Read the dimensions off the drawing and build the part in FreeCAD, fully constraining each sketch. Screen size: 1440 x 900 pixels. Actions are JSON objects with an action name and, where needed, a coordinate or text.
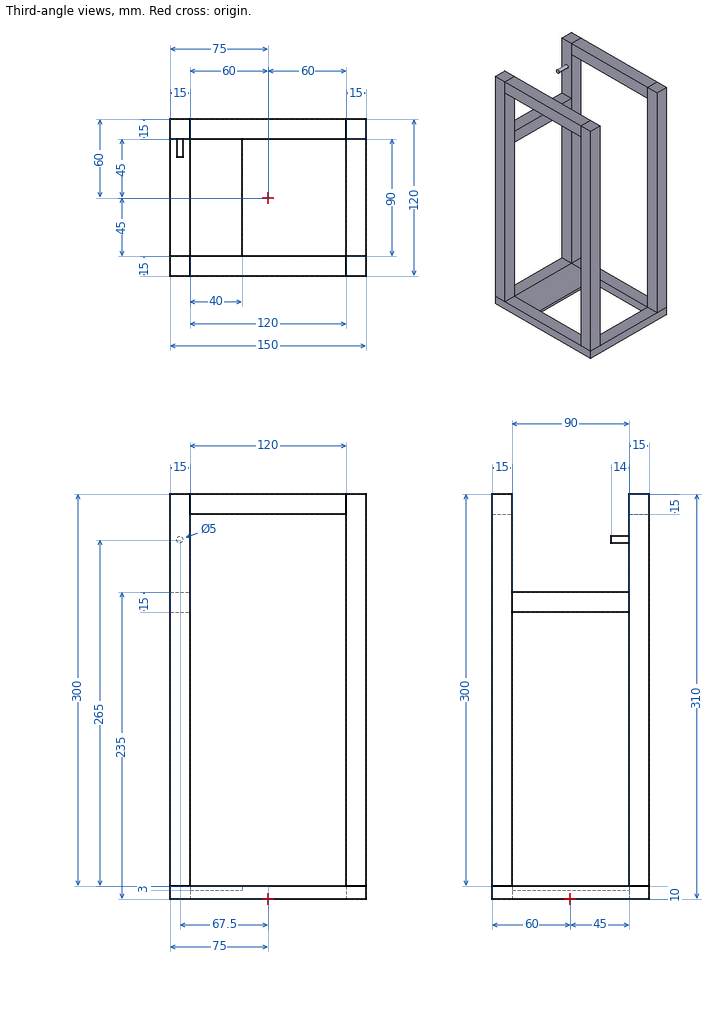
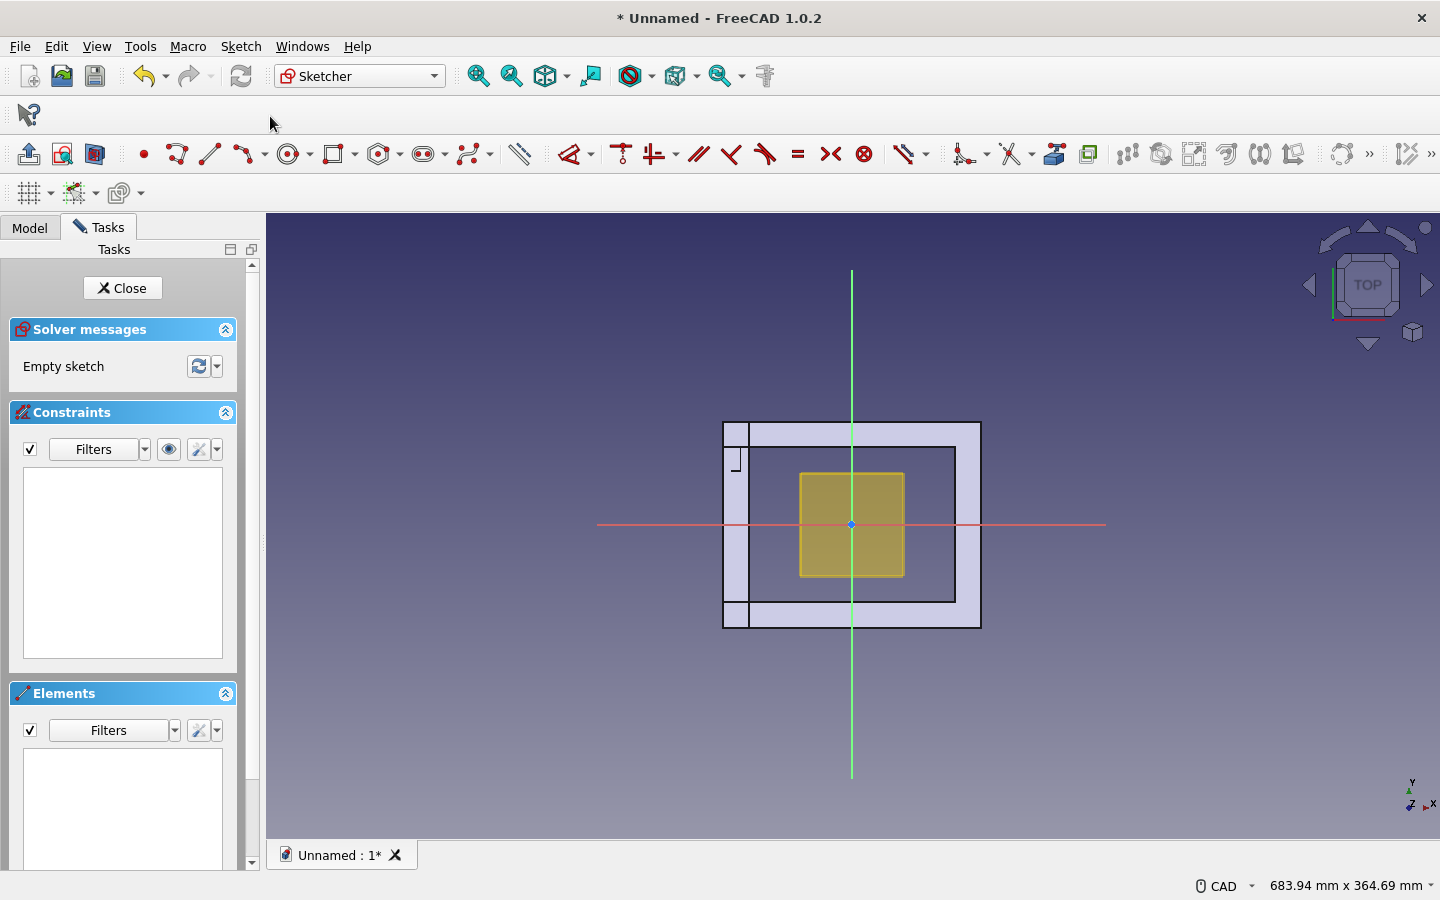
{"action": "scroll", "coordinate": [980, 429], "scroll_direction": "up", "scroll_amount": 14}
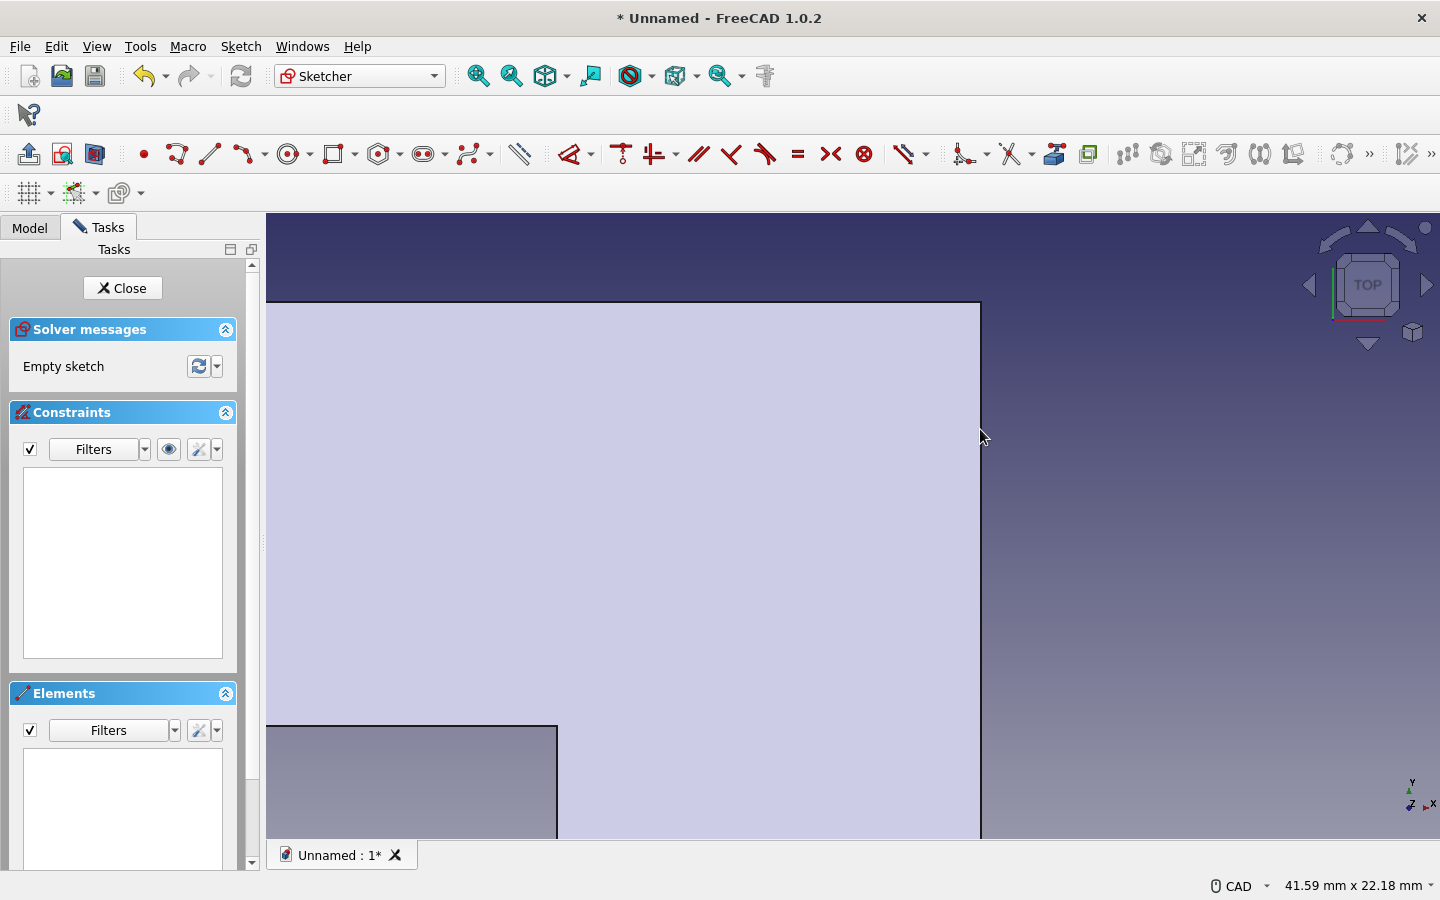
{"action": "left_click", "coordinate": [332, 154]}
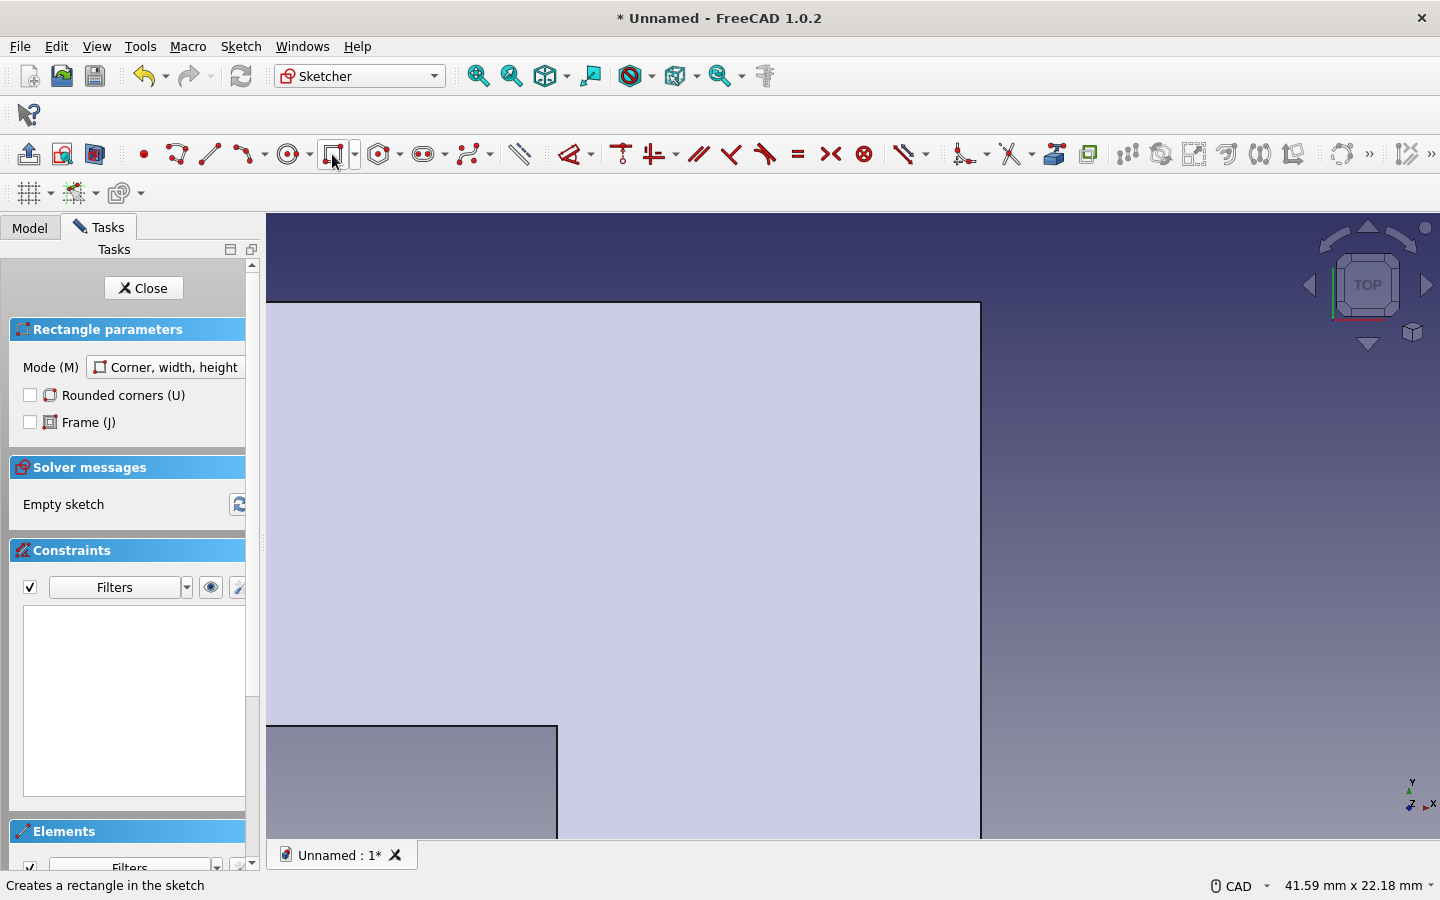
{"action": "left_click", "coordinate": [557, 302]}
{"action": "left_click", "coordinate": [981, 726]}
{"action": "key", "text": "Escape"}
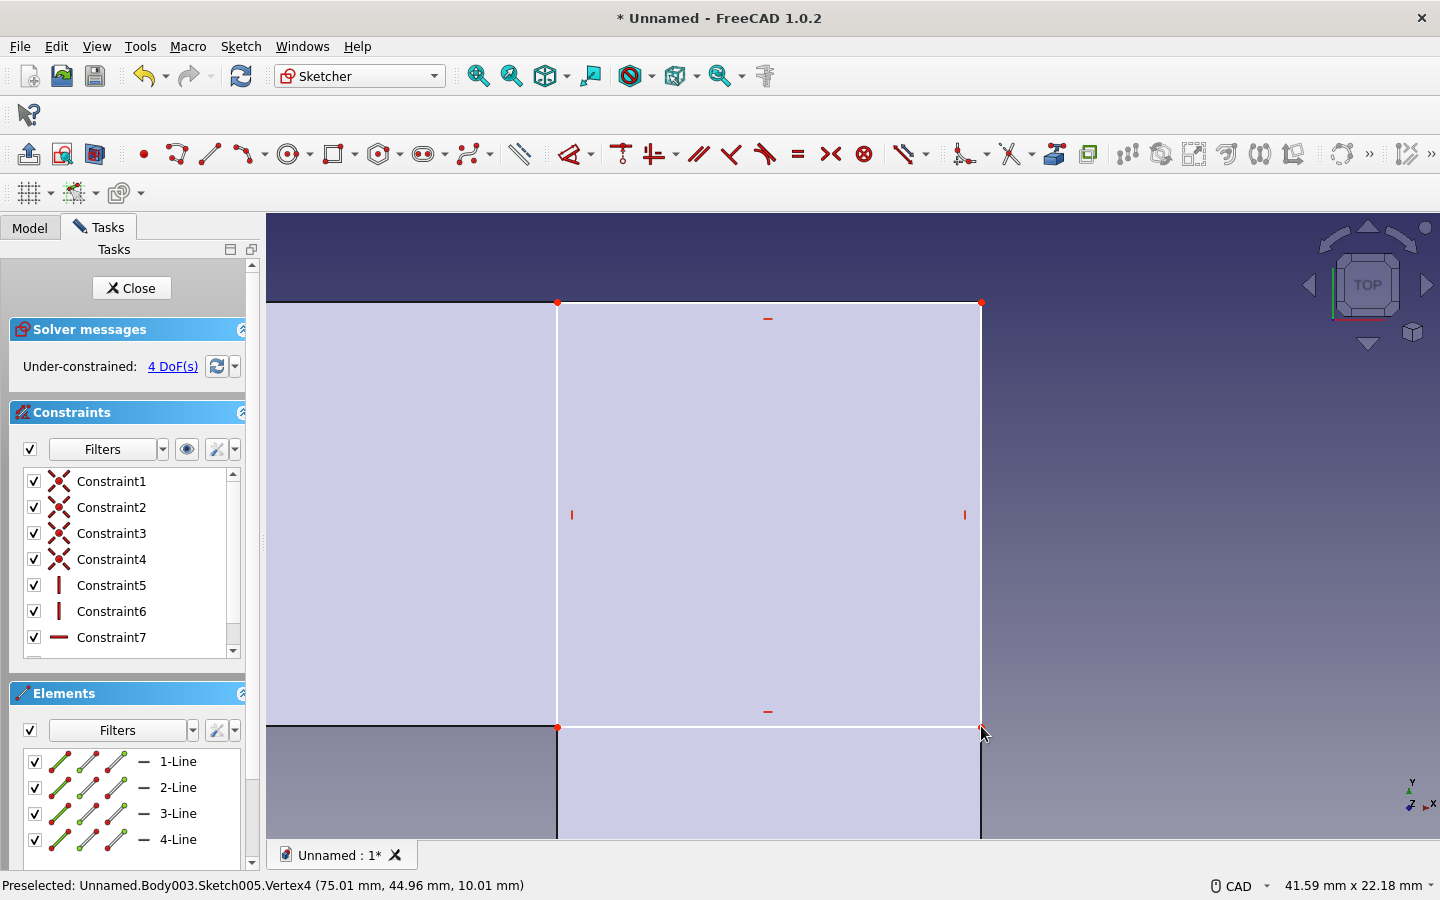
{"action": "left_click", "coordinate": [568, 154]}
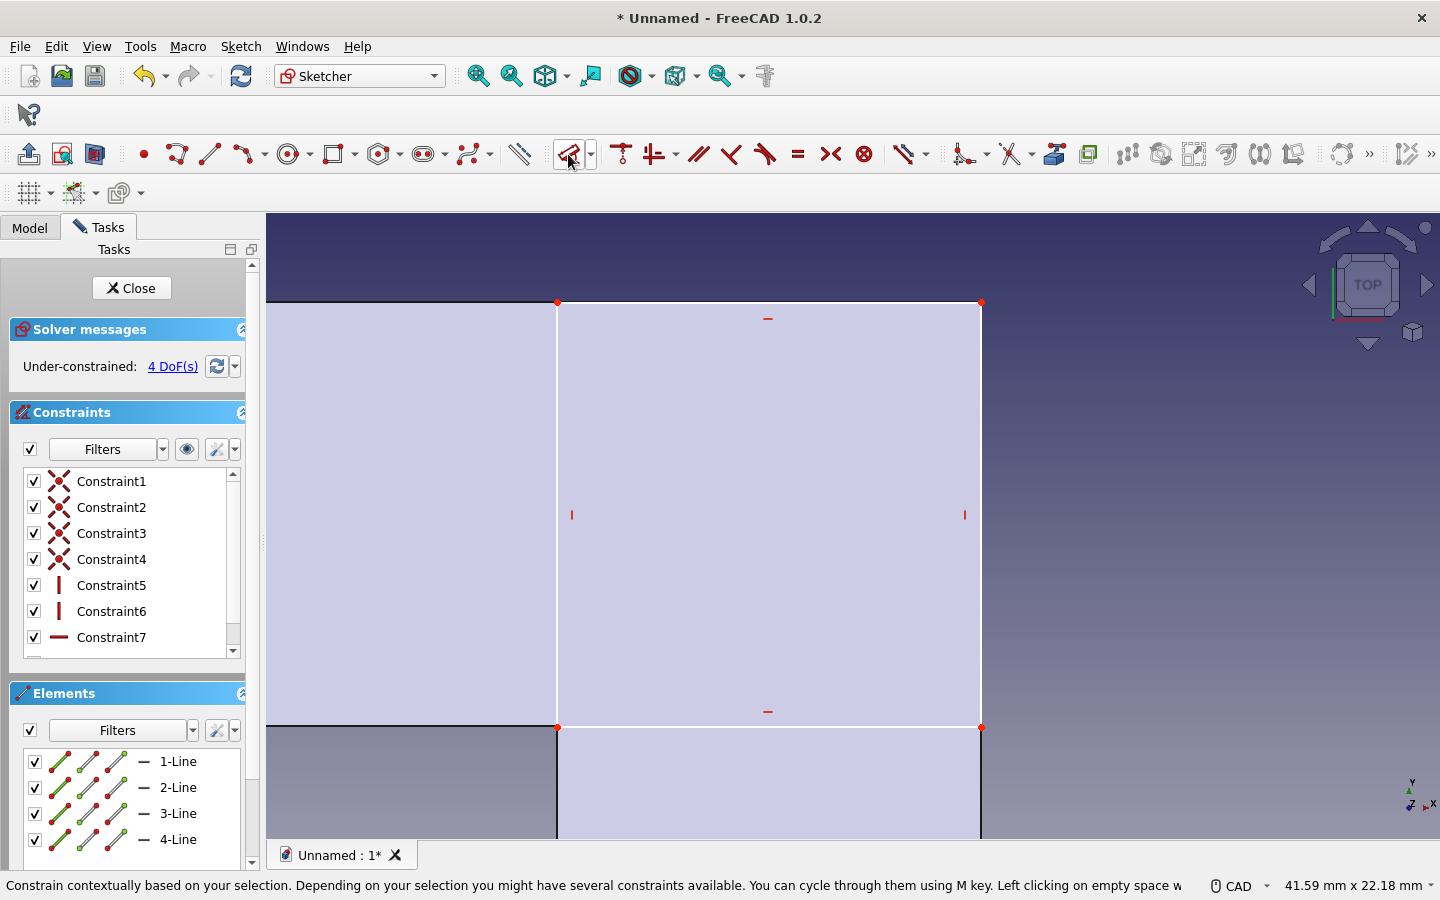
{"action": "left_click", "coordinate": [557, 430]}
{"action": "left_click", "coordinate": [523, 515]}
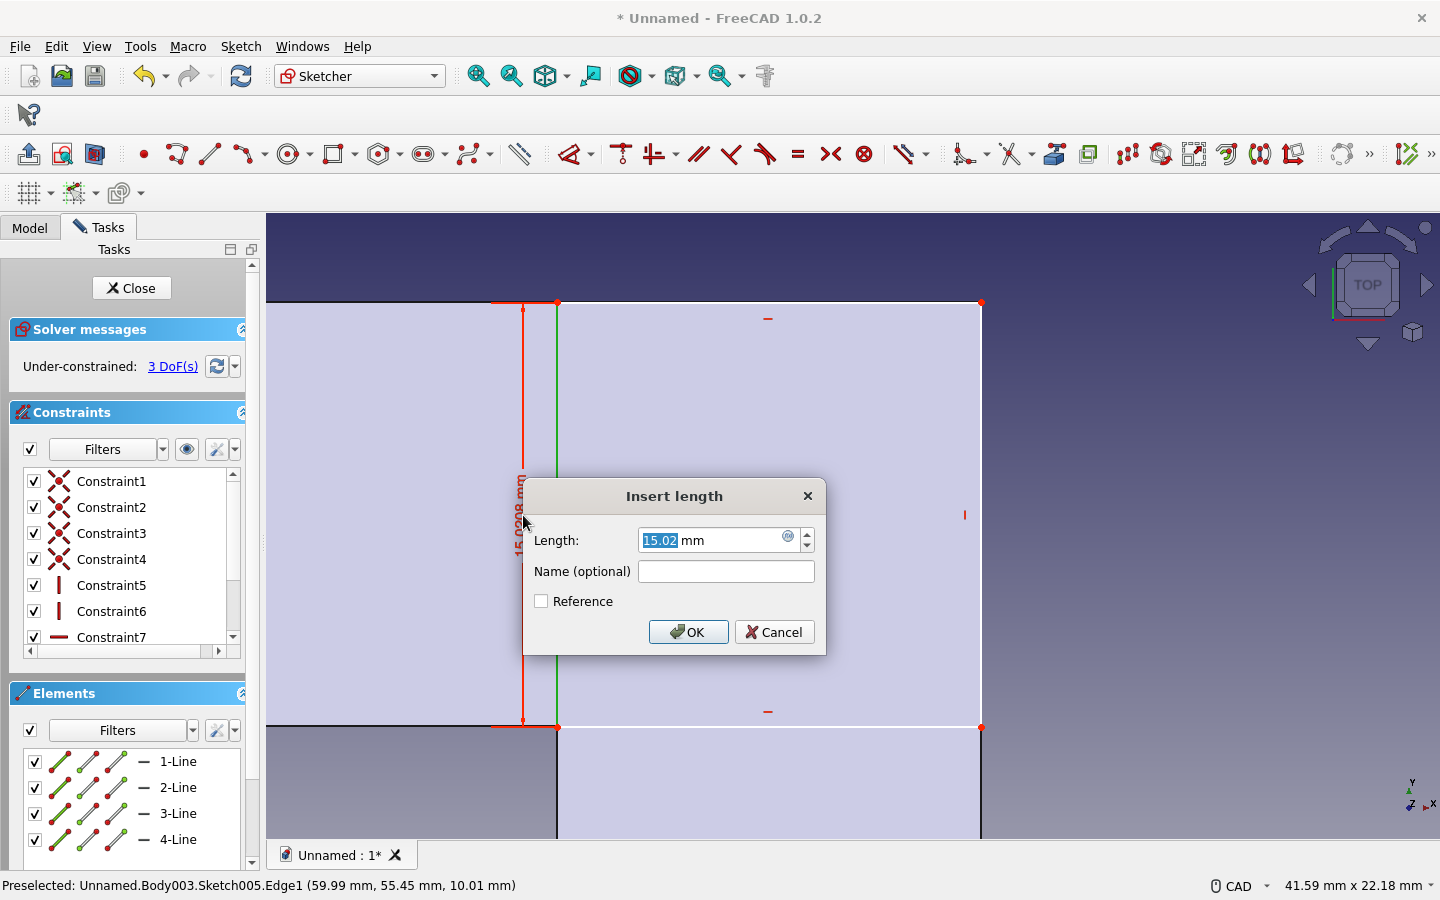
{"action": "type", "text": "15"}
{"action": "key", "text": "Return"}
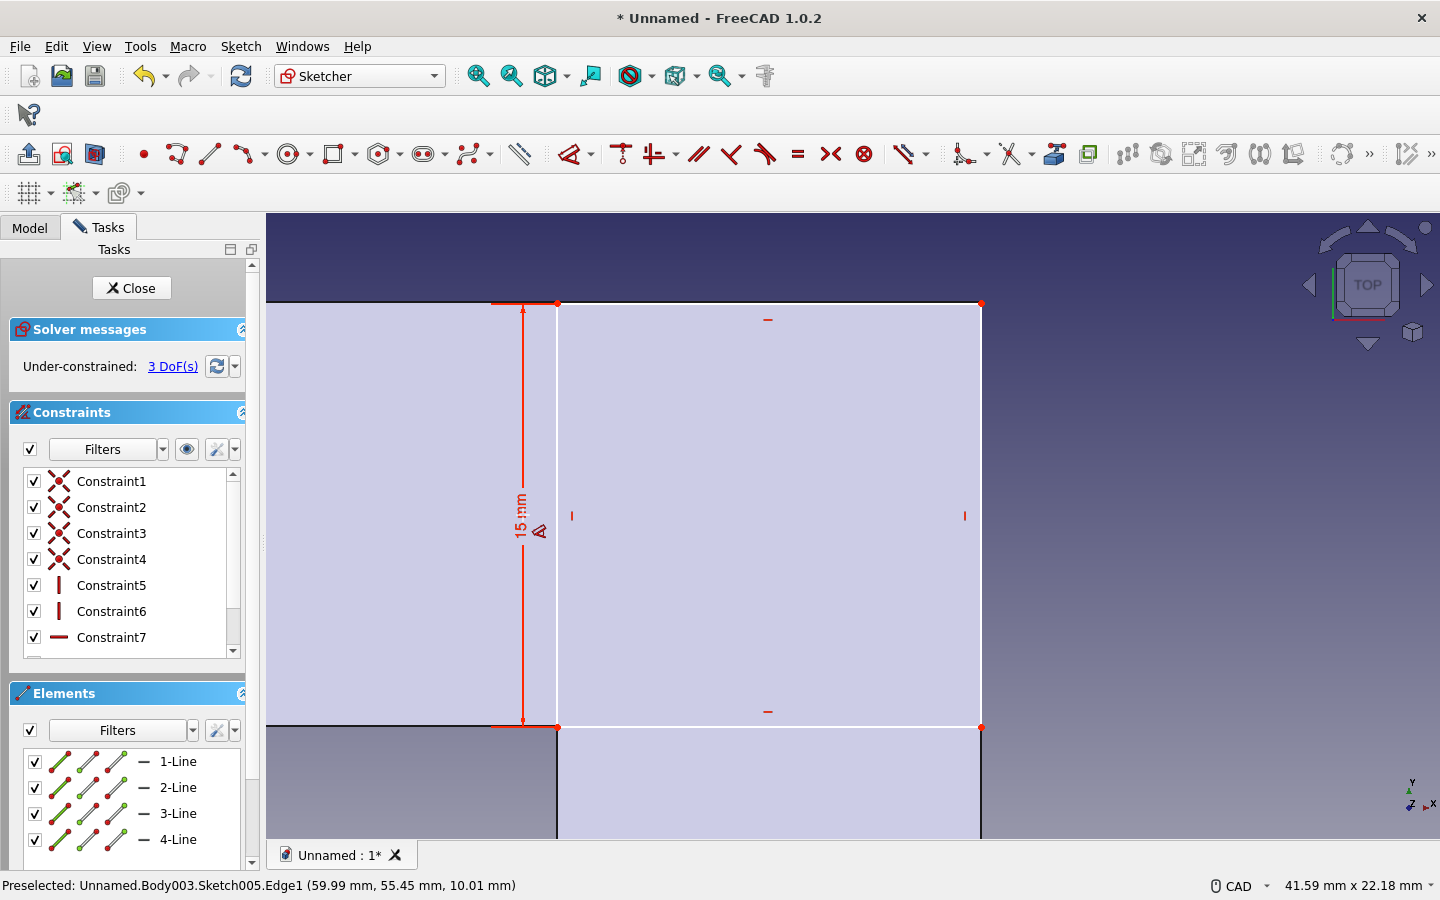
{"action": "left_click", "coordinate": [684, 727]}
{"action": "left_click", "coordinate": [769, 761]}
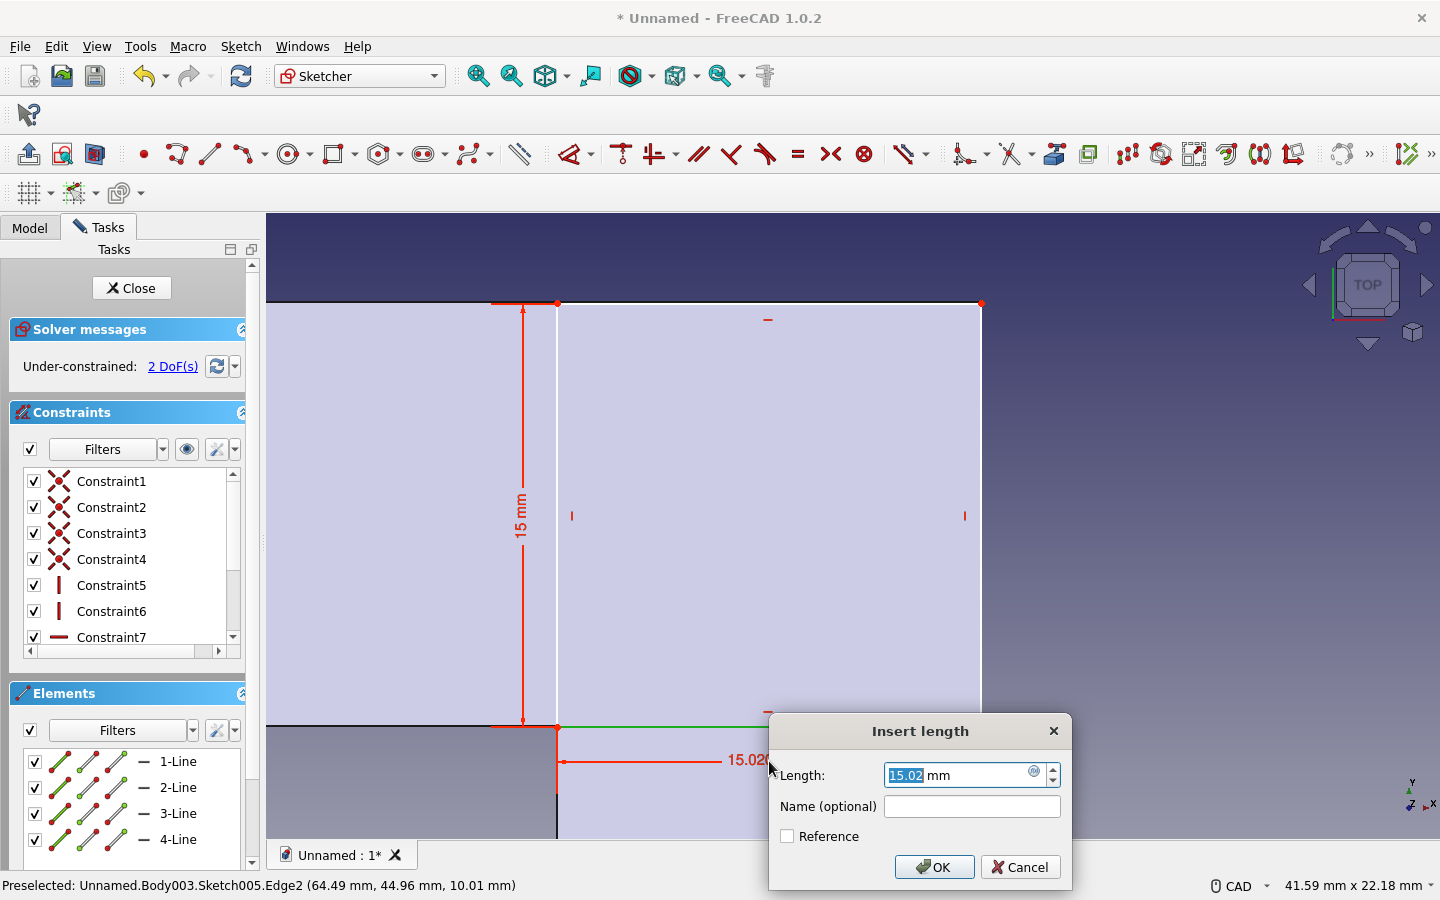
{"action": "type", "text": "15"}
{"action": "key", "text": "Return"}